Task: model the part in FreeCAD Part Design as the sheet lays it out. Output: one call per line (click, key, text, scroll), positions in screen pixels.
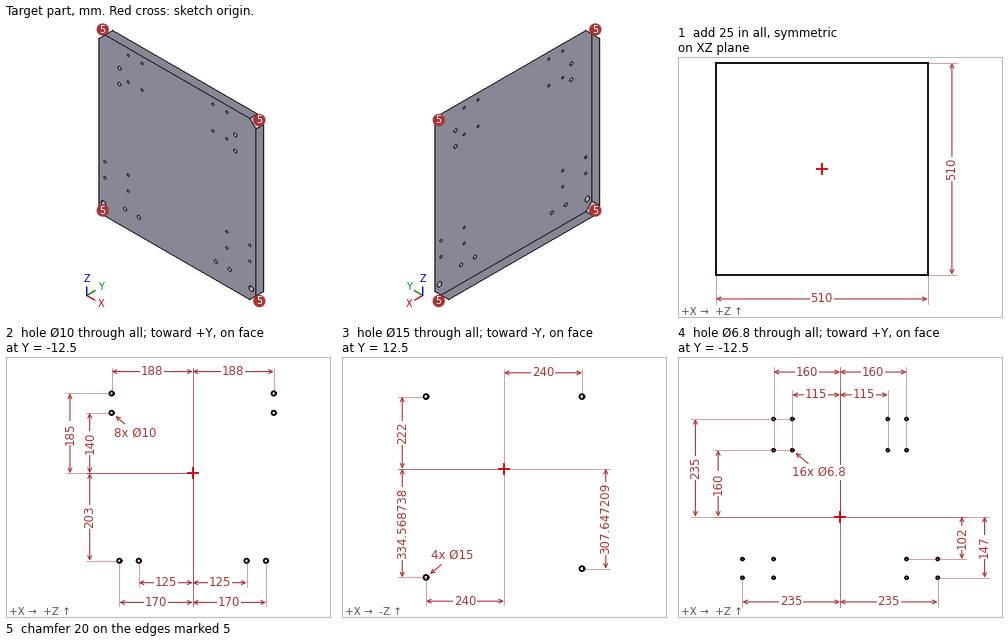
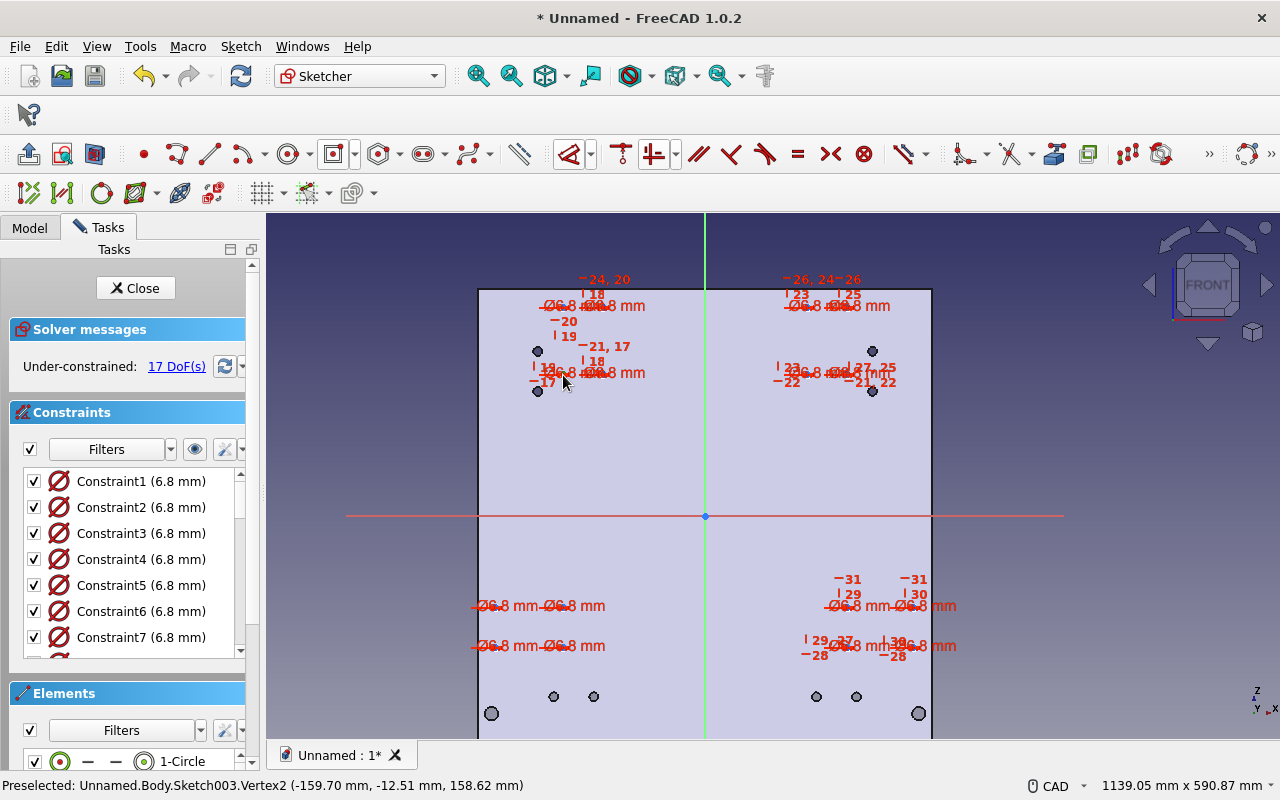
click(563, 648)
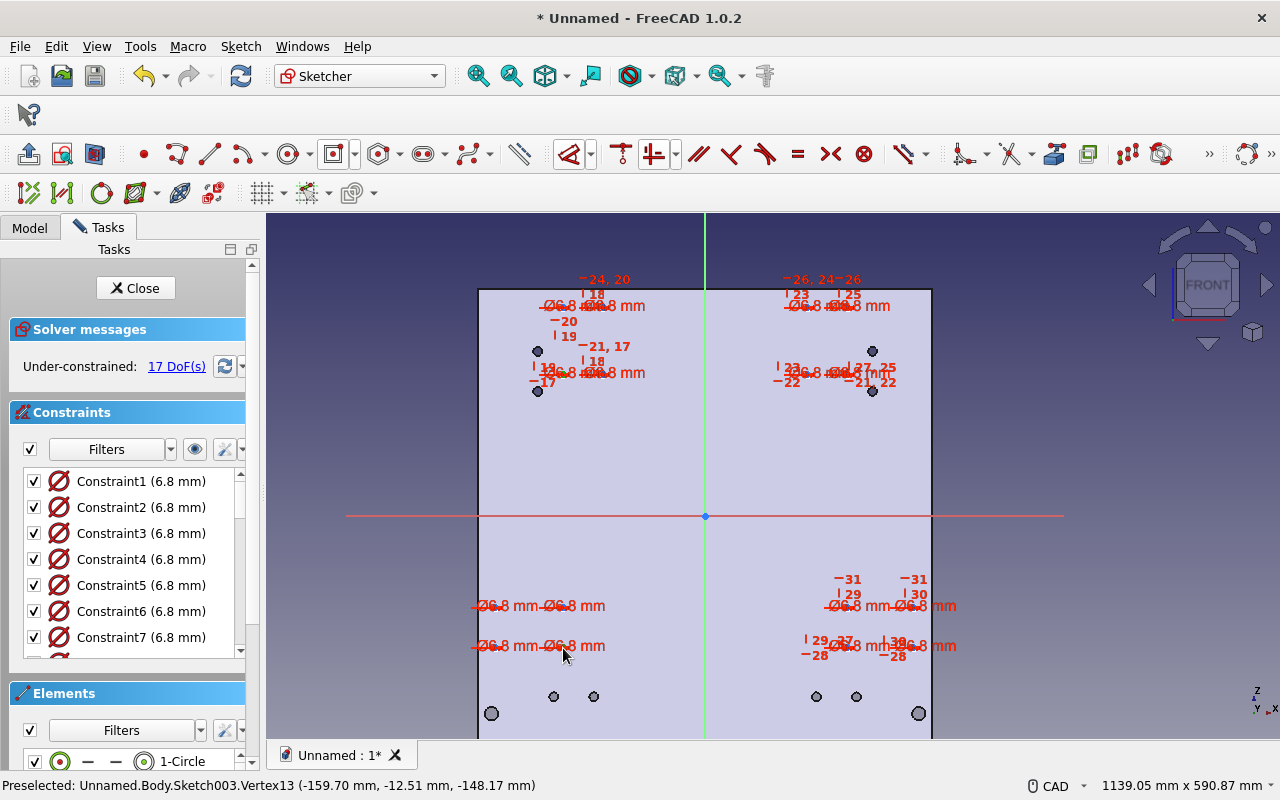
key(v)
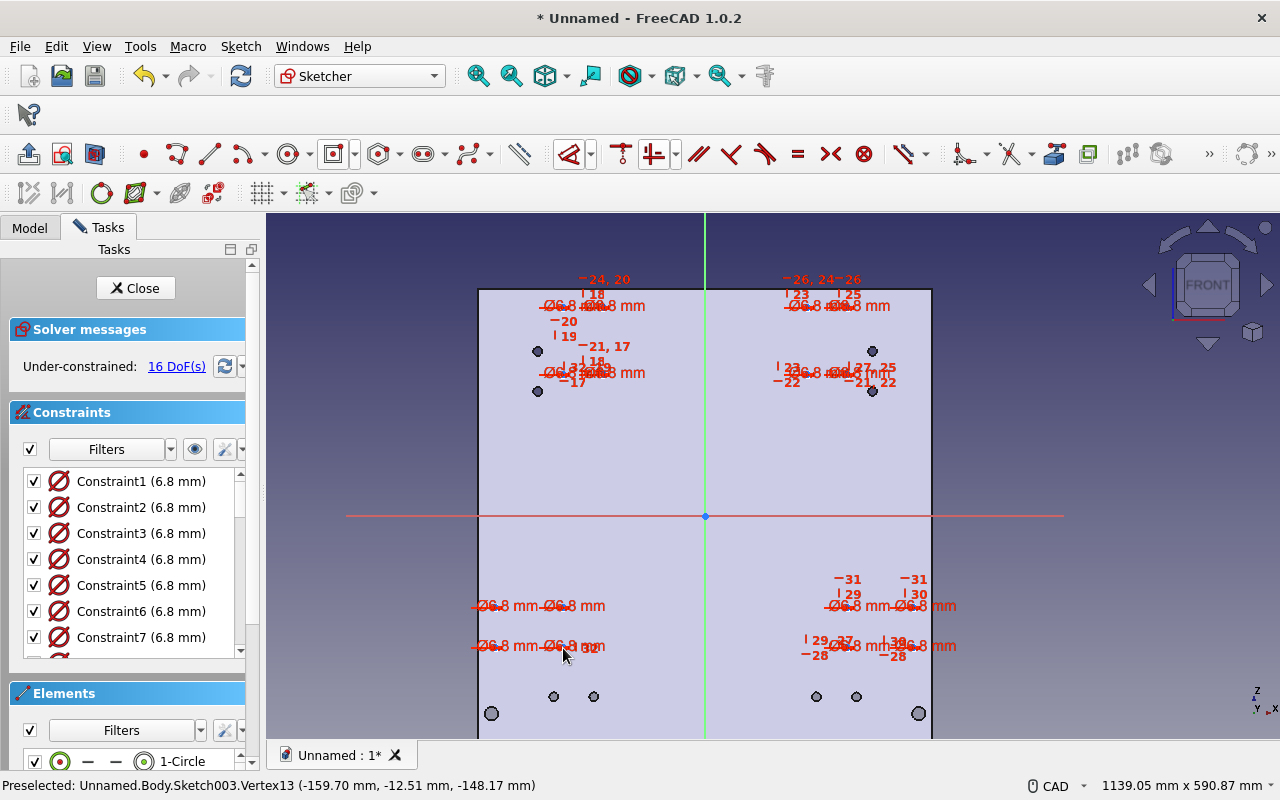
click(848, 648)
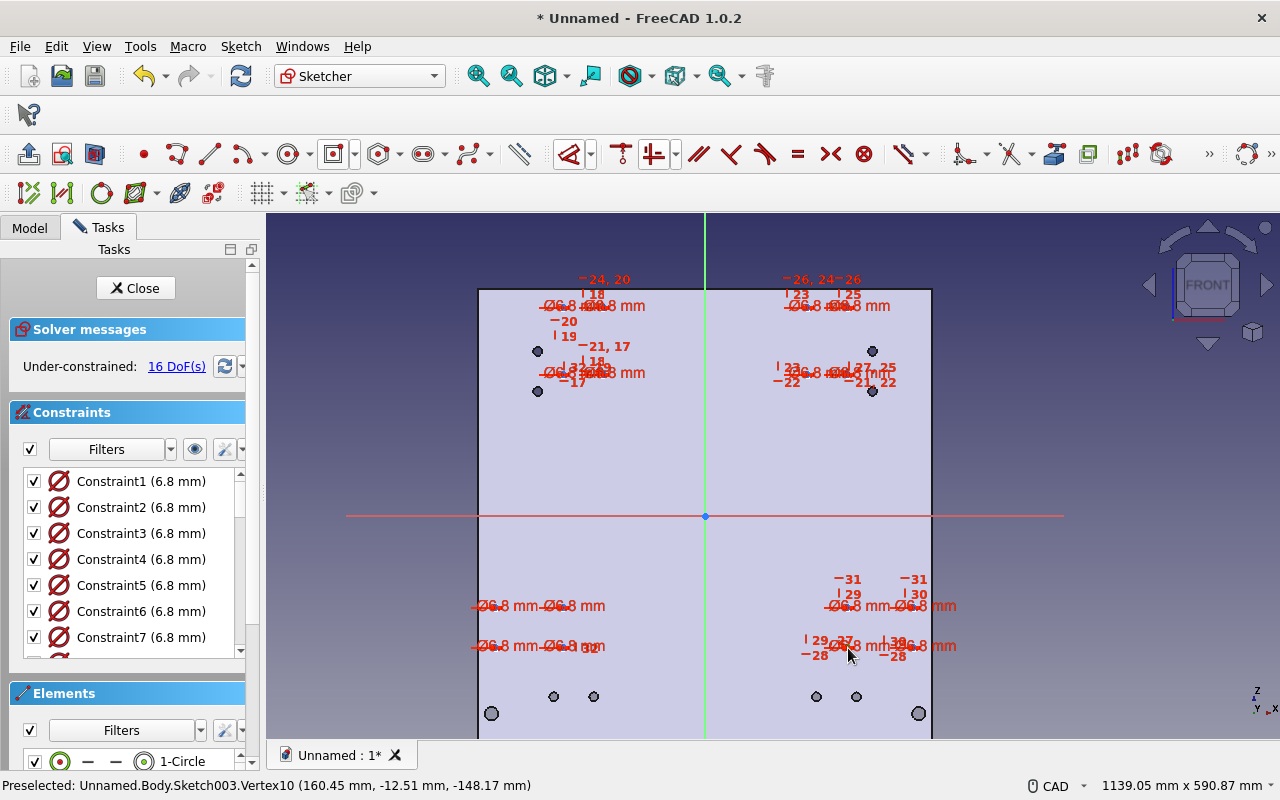
click(563, 648)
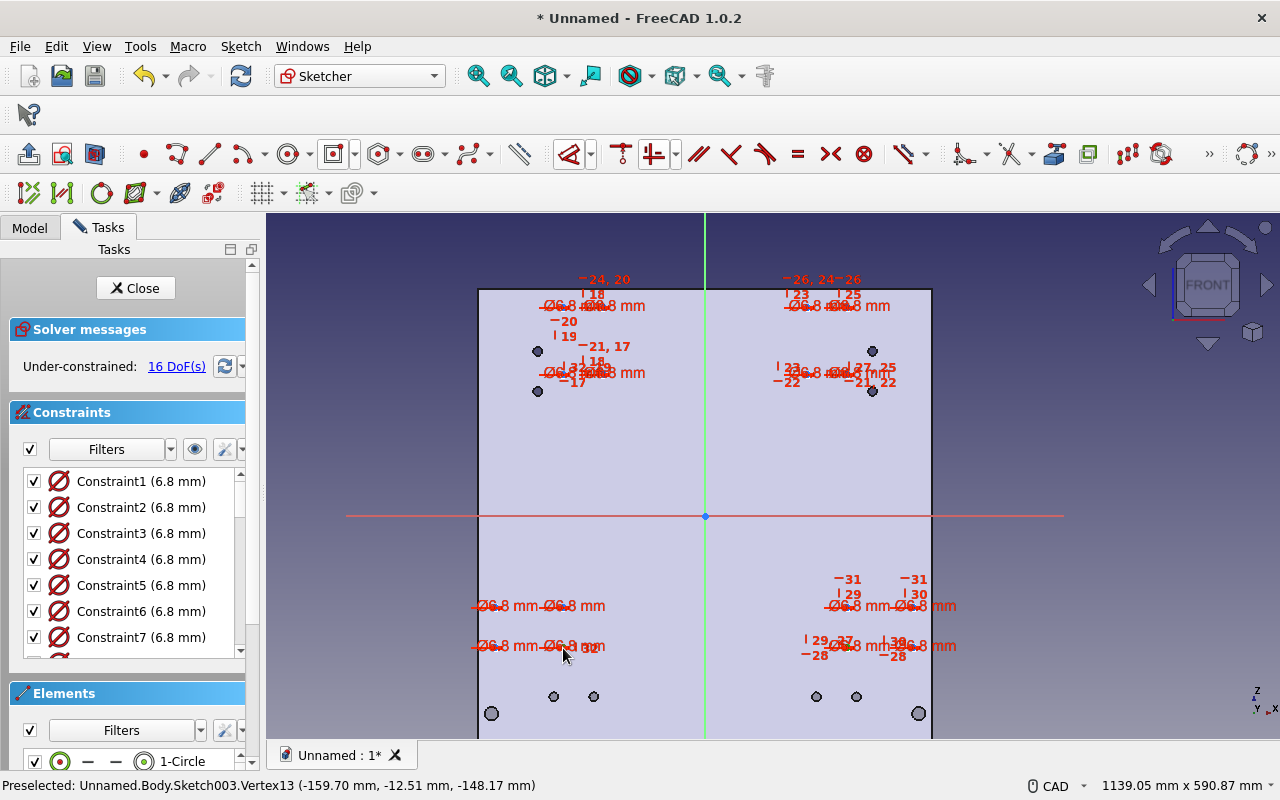
click(676, 154)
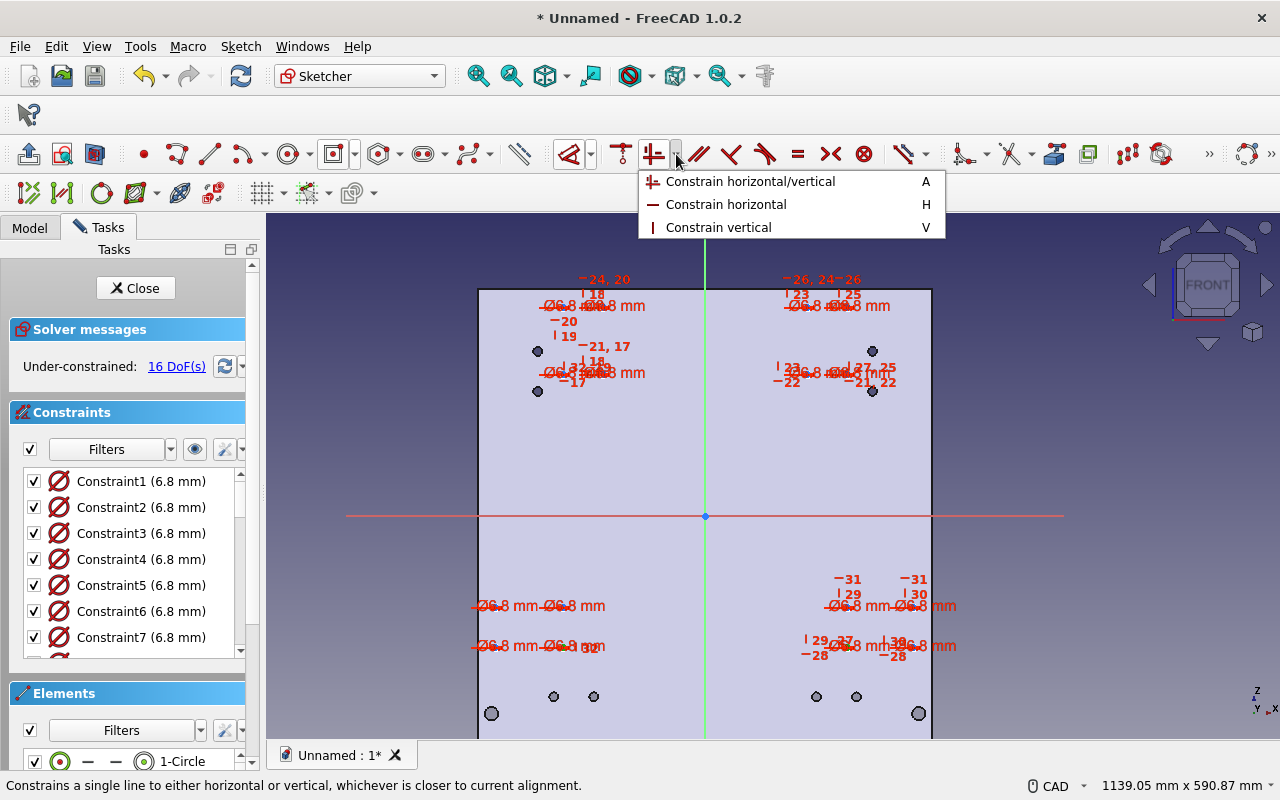
click(792, 204)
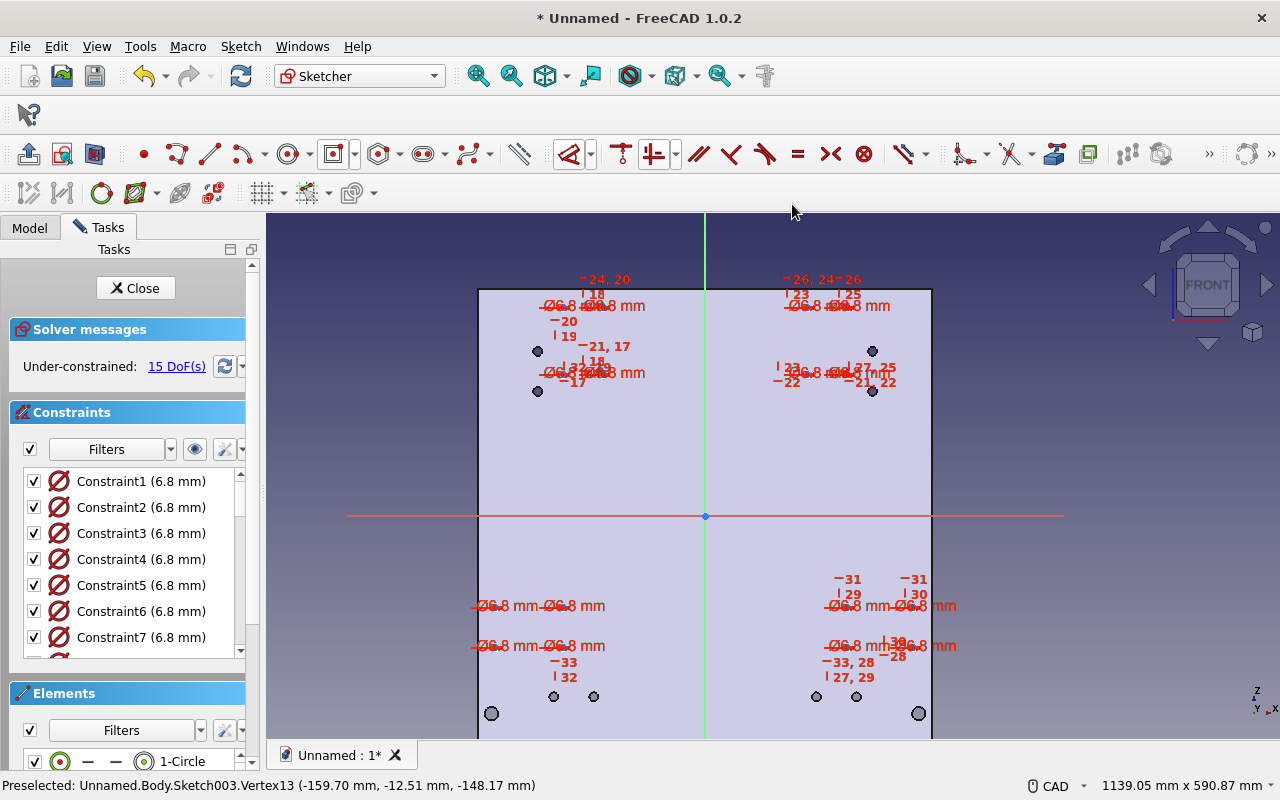
click(563, 648)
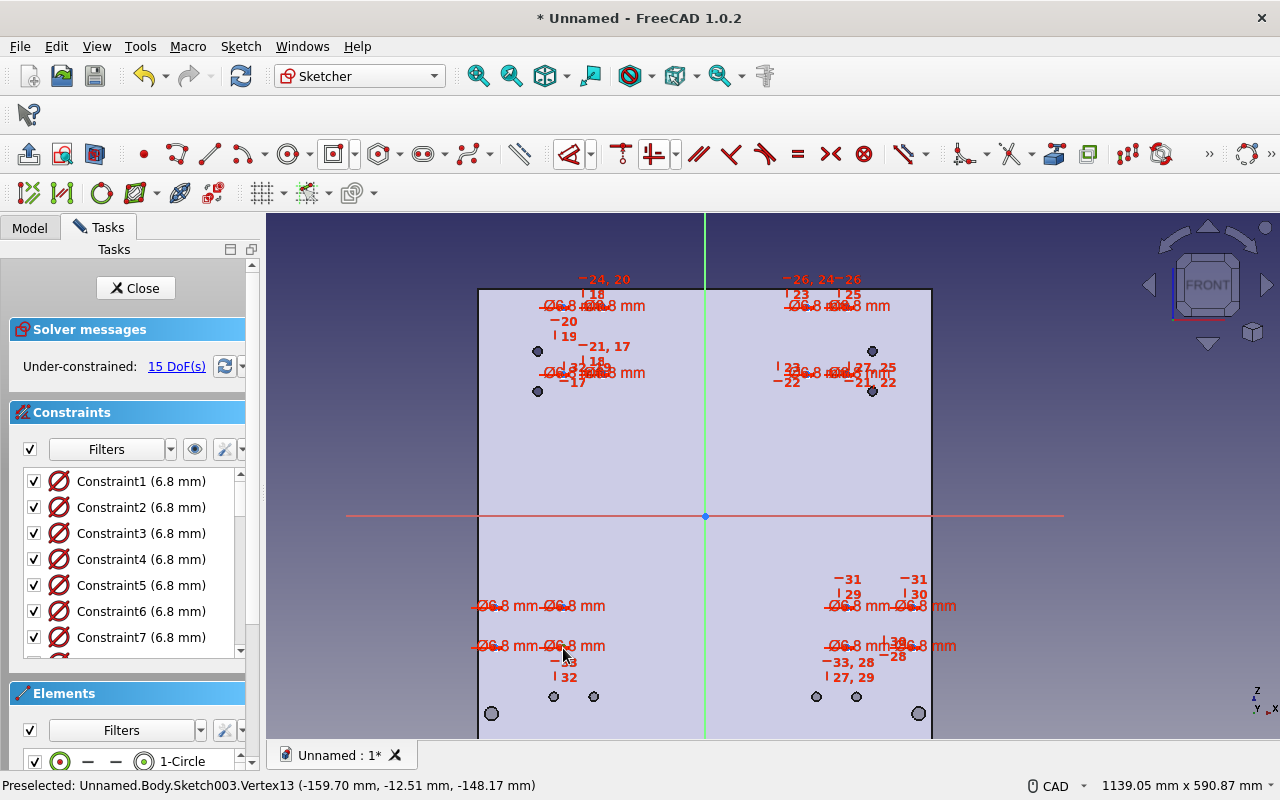
click(496, 648)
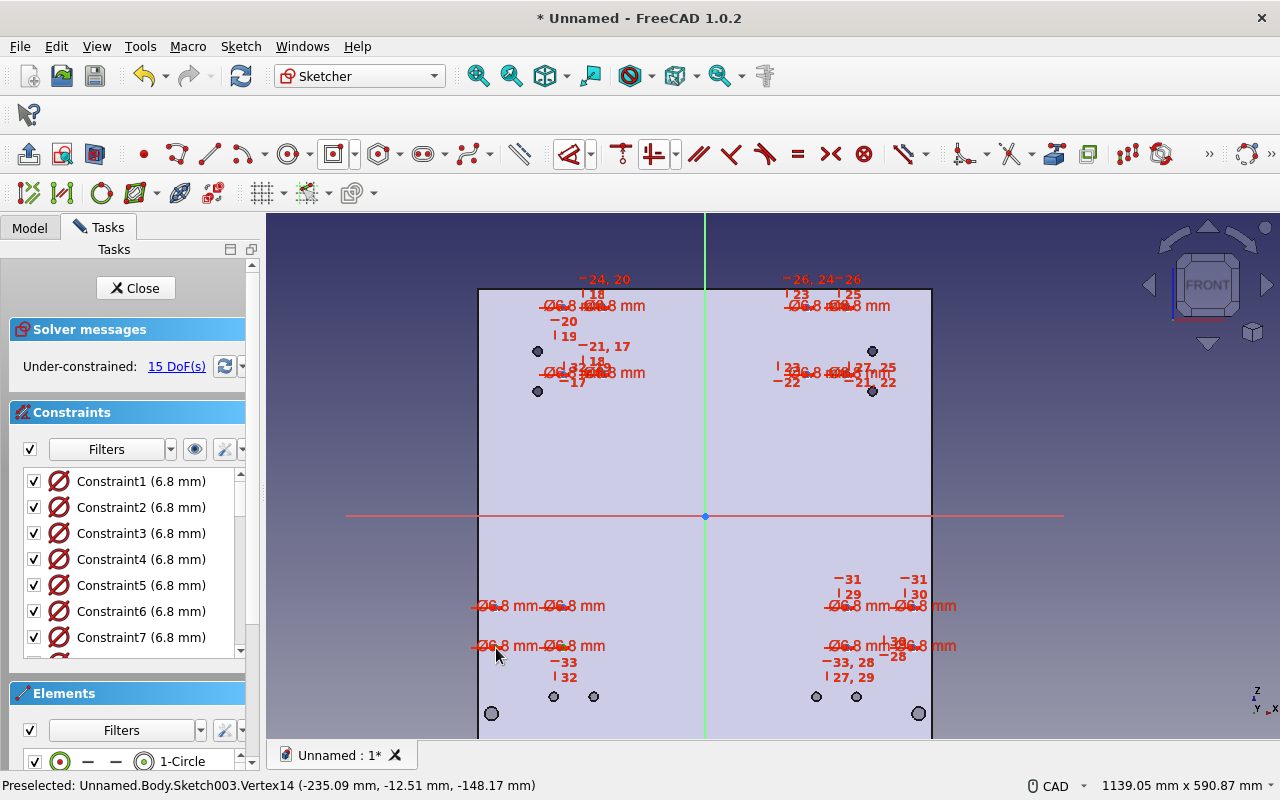
key(h)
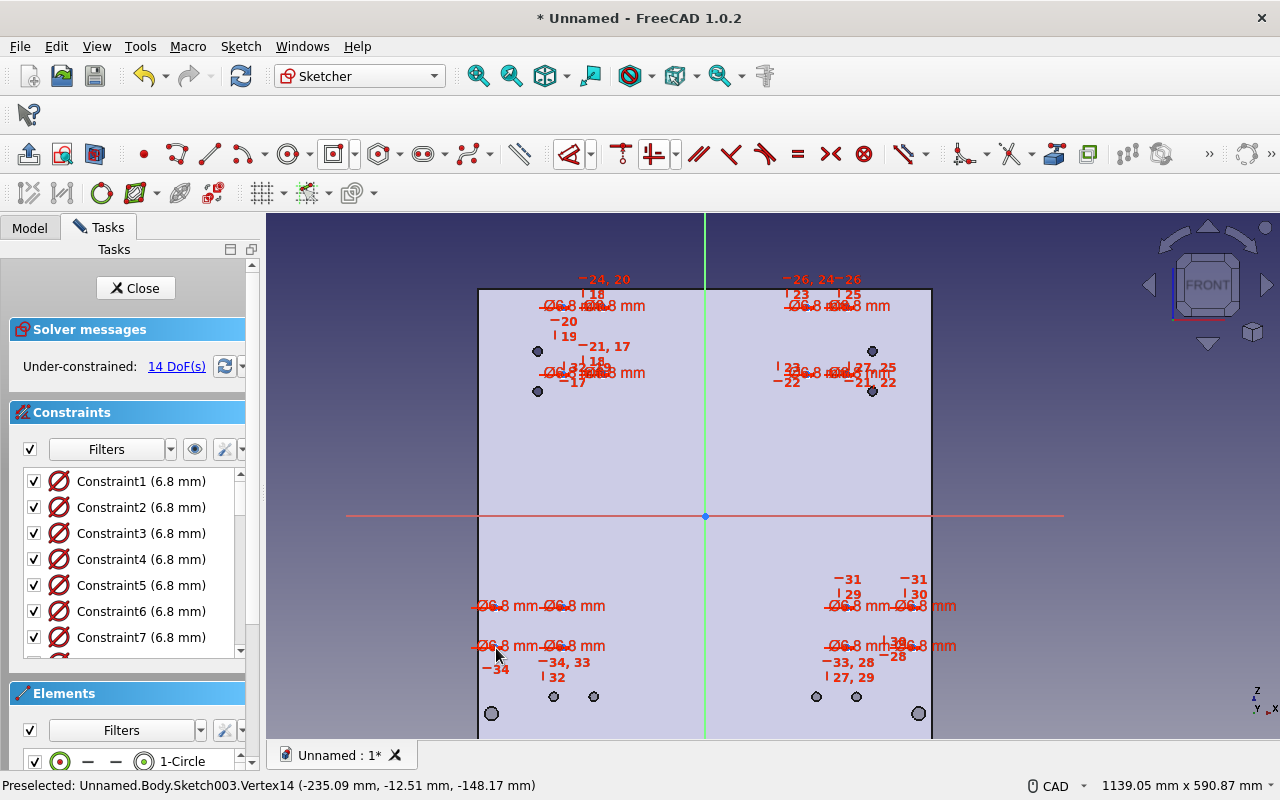
click(496, 648)